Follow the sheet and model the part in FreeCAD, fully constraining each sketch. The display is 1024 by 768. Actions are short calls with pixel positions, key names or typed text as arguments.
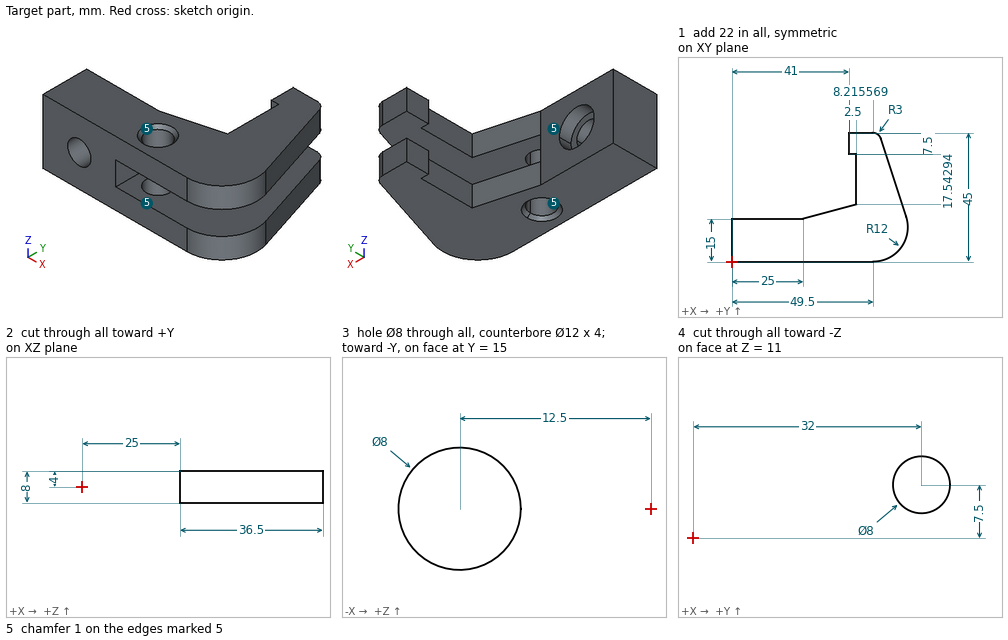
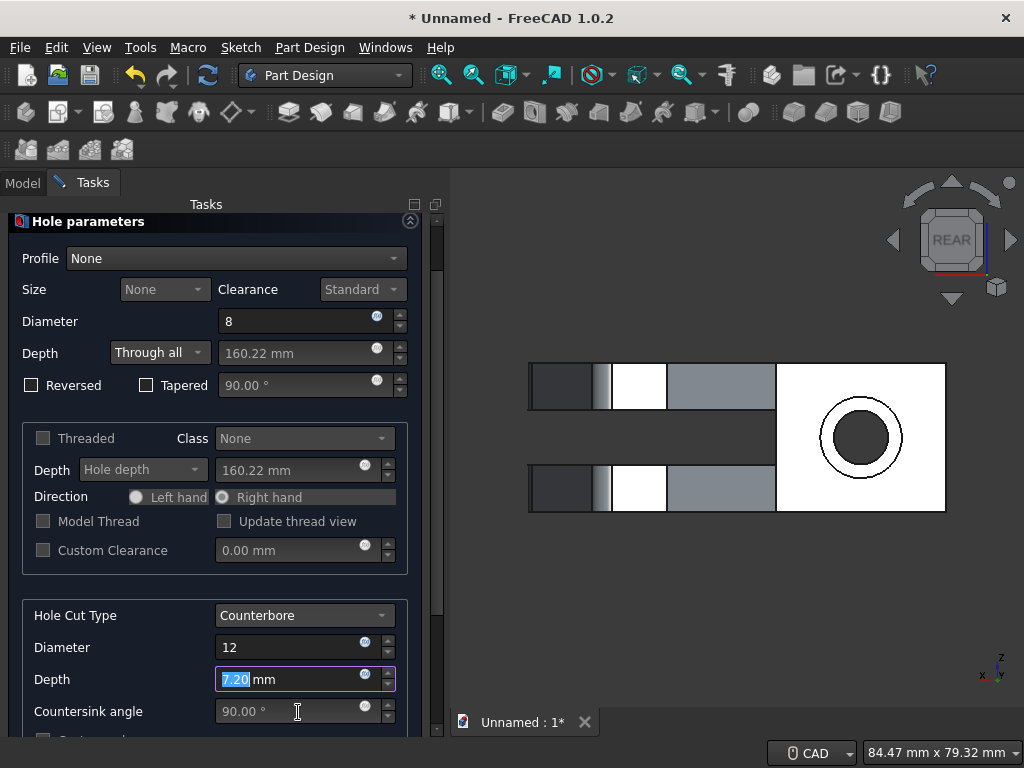
text(4)
key(Tab)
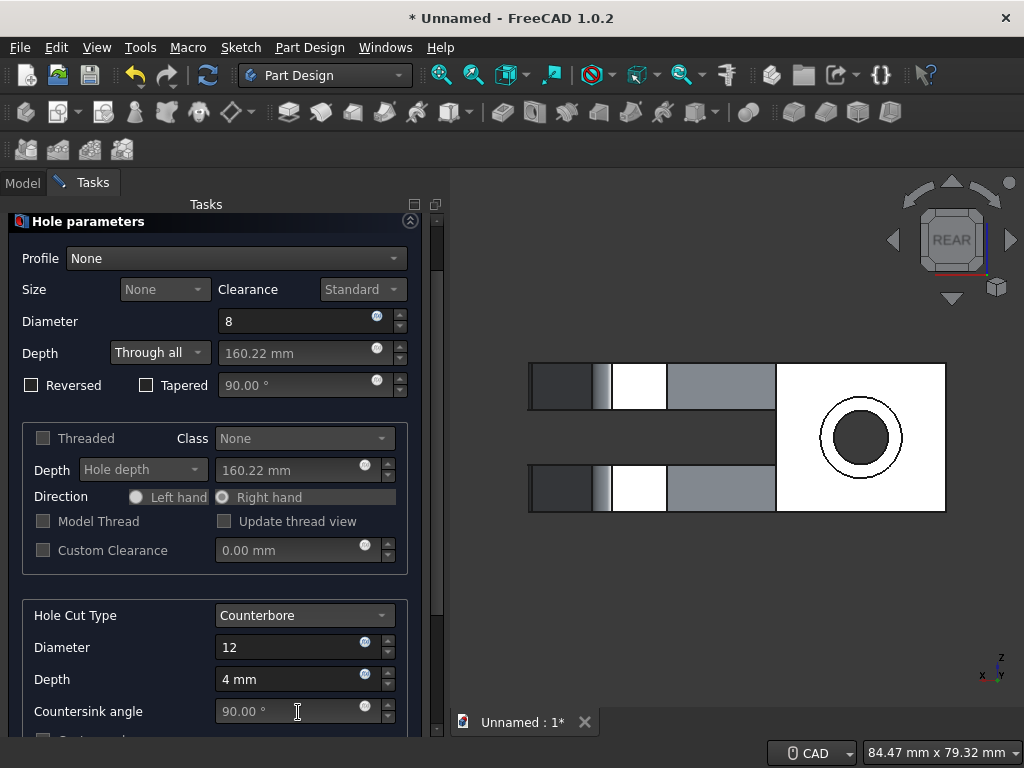
scroll(437, 475, up, 2)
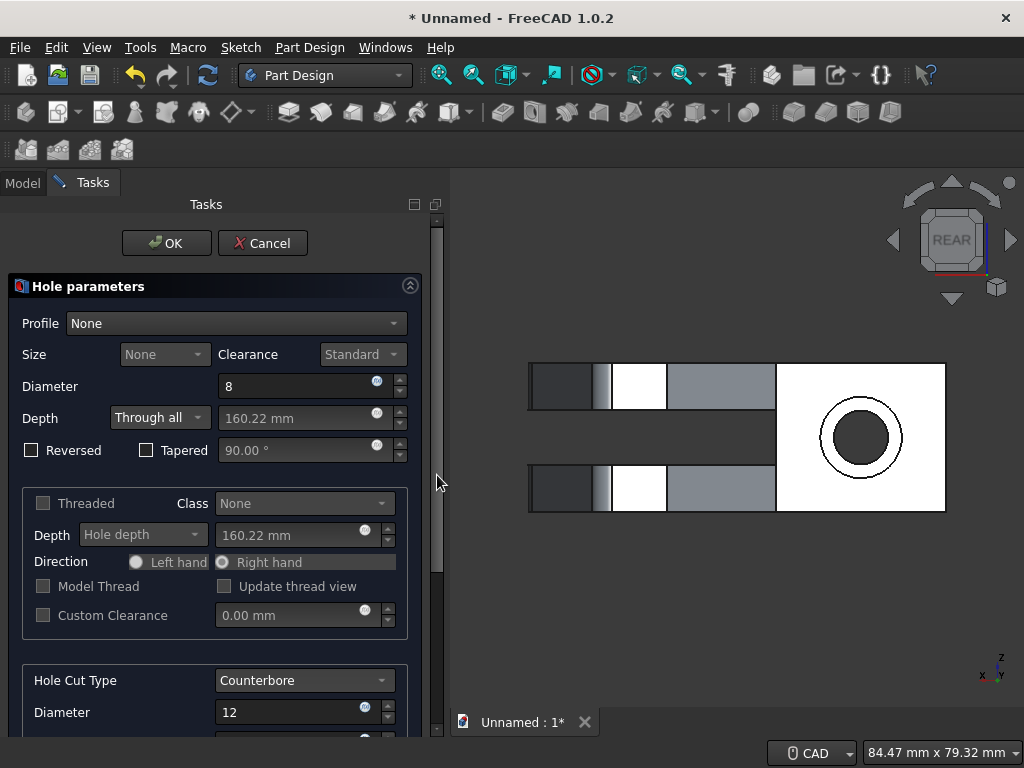
click(167, 243)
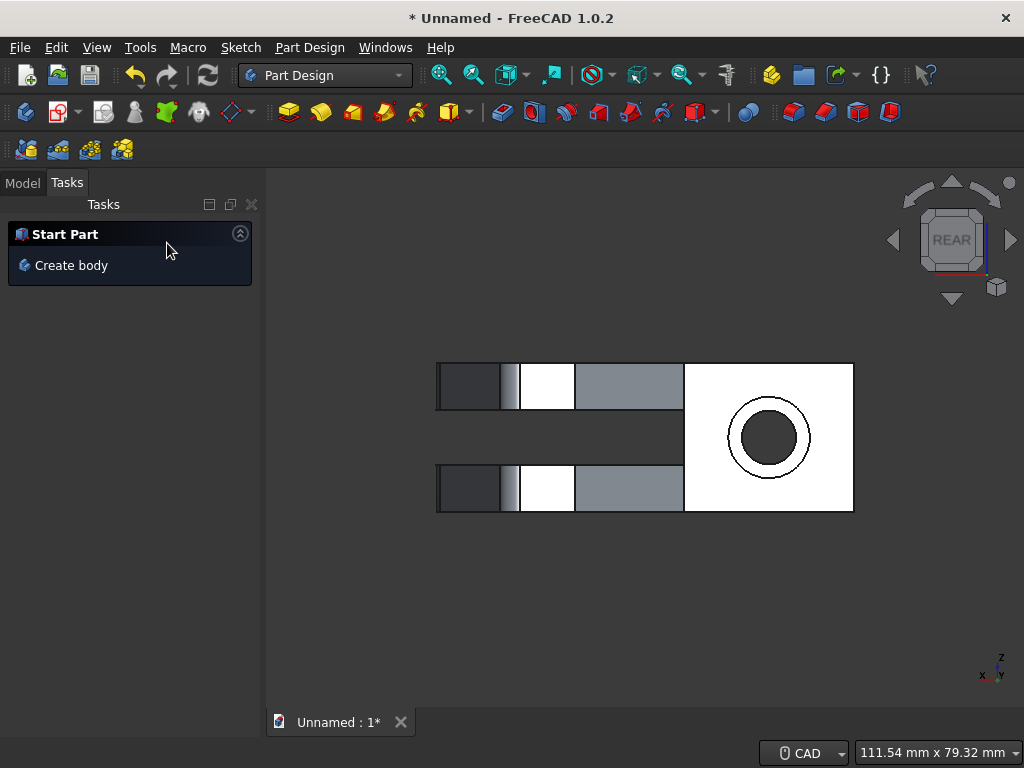
key(0)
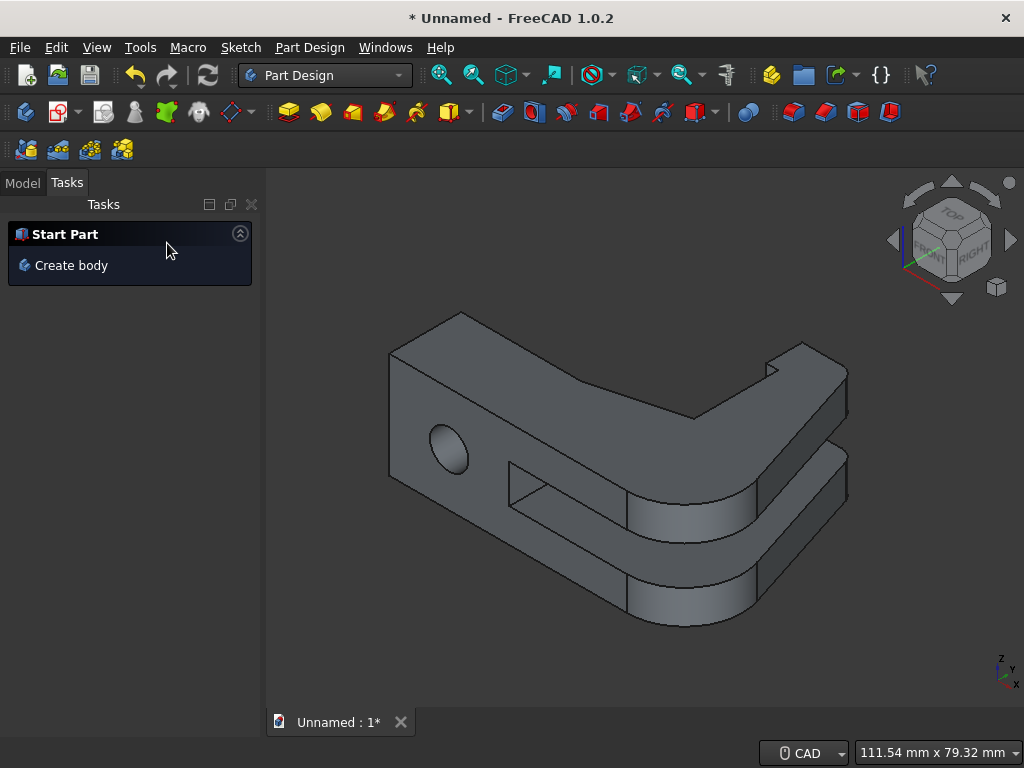
click(668, 460)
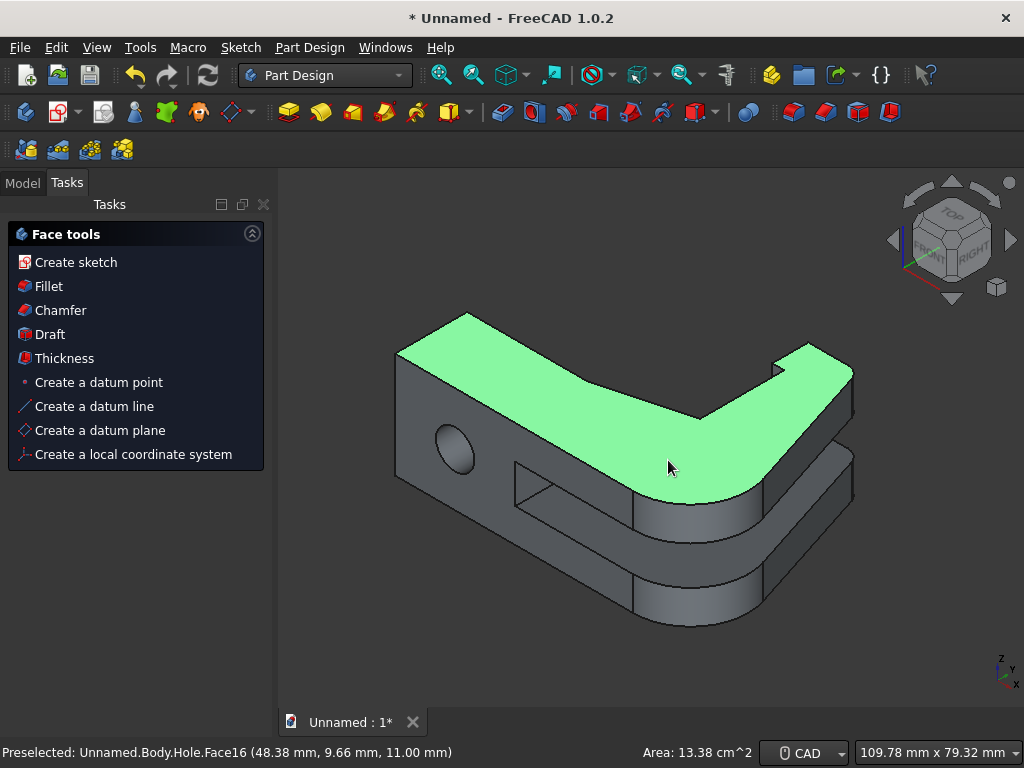
click(58, 112)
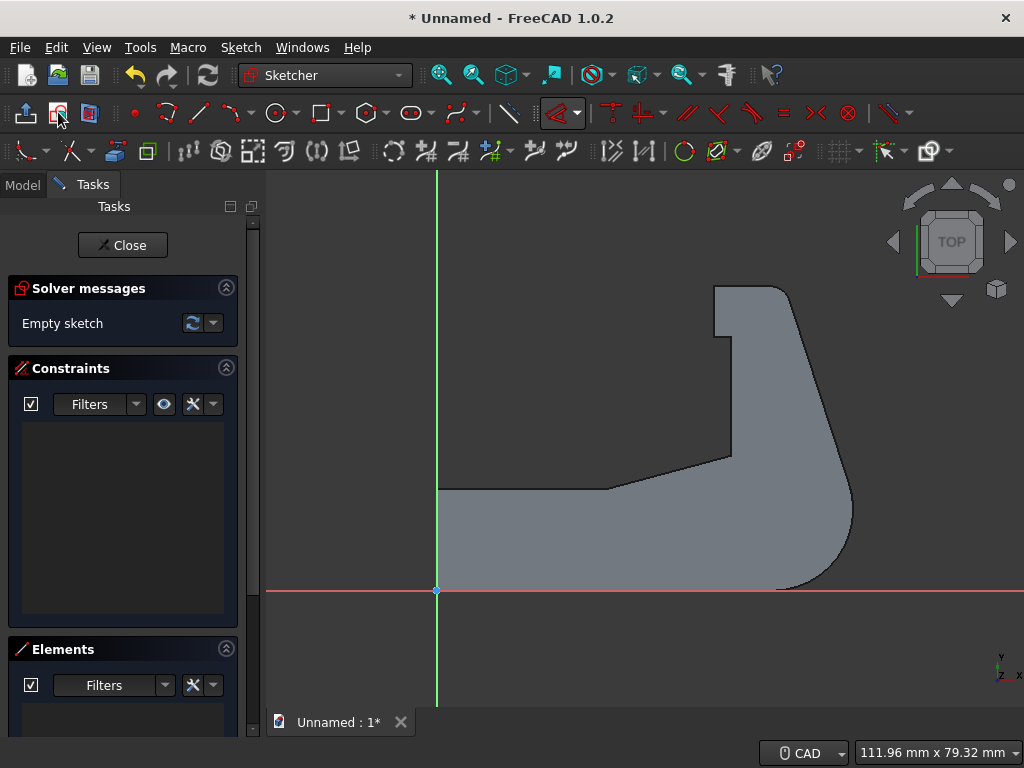
scroll(669, 560, up, 9)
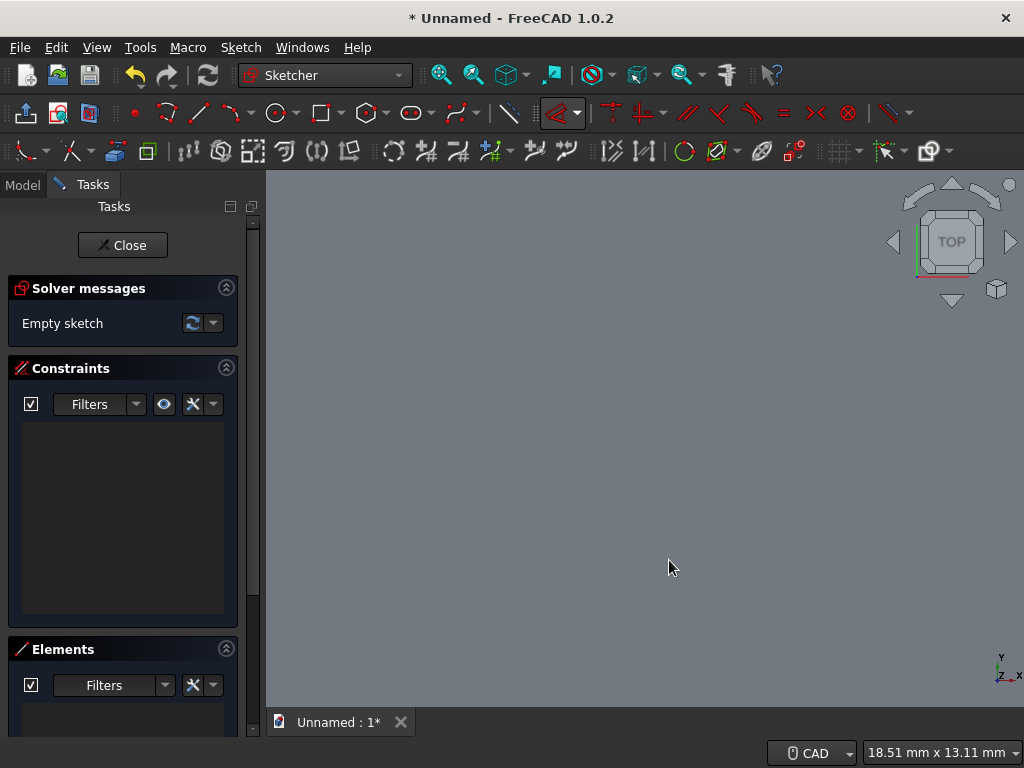
key(g)
key(c)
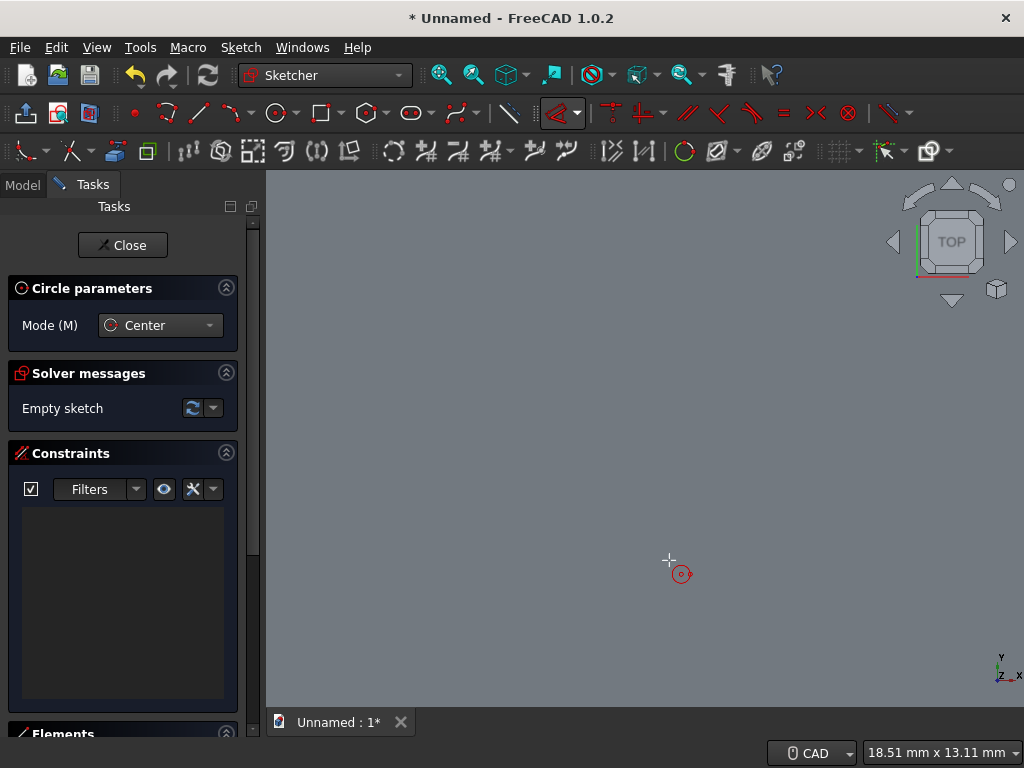
click(572, 436)
click(688, 320)
key(Escape)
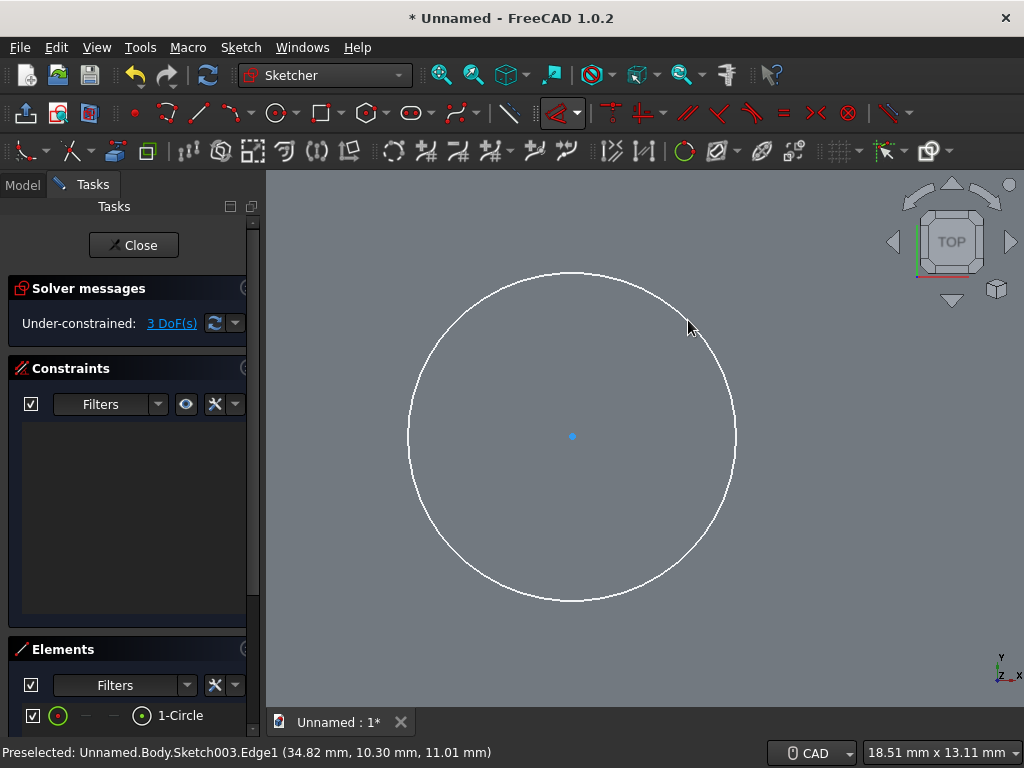
click(688, 321)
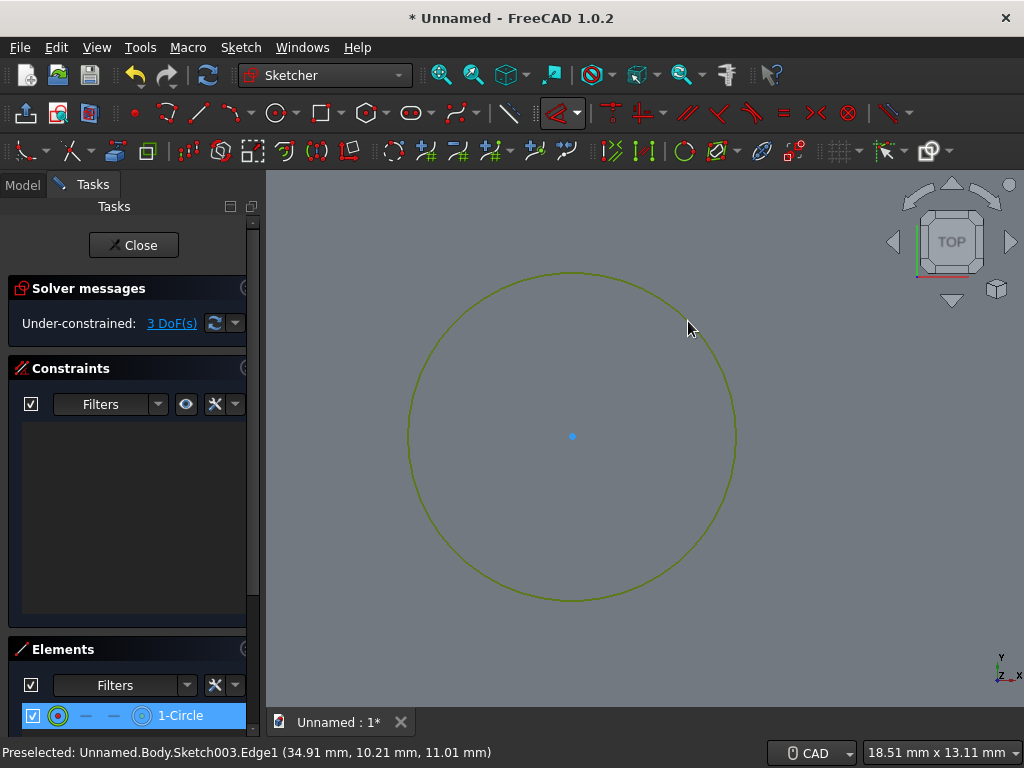
key(k)
key(o)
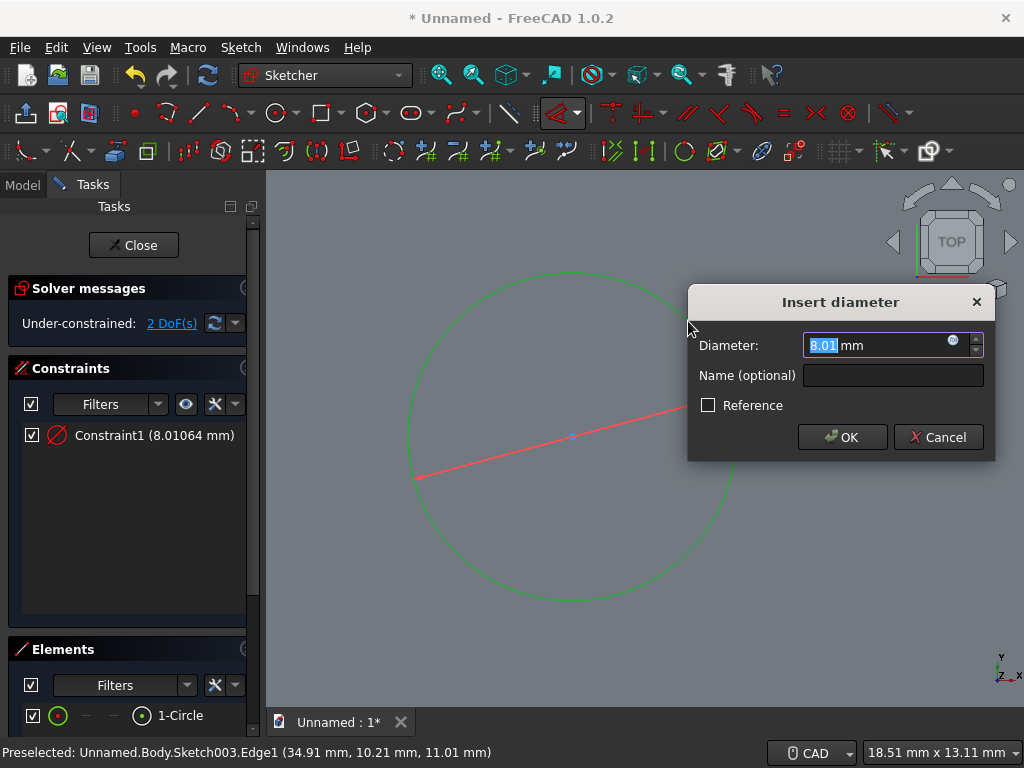
text(8)
key(Return)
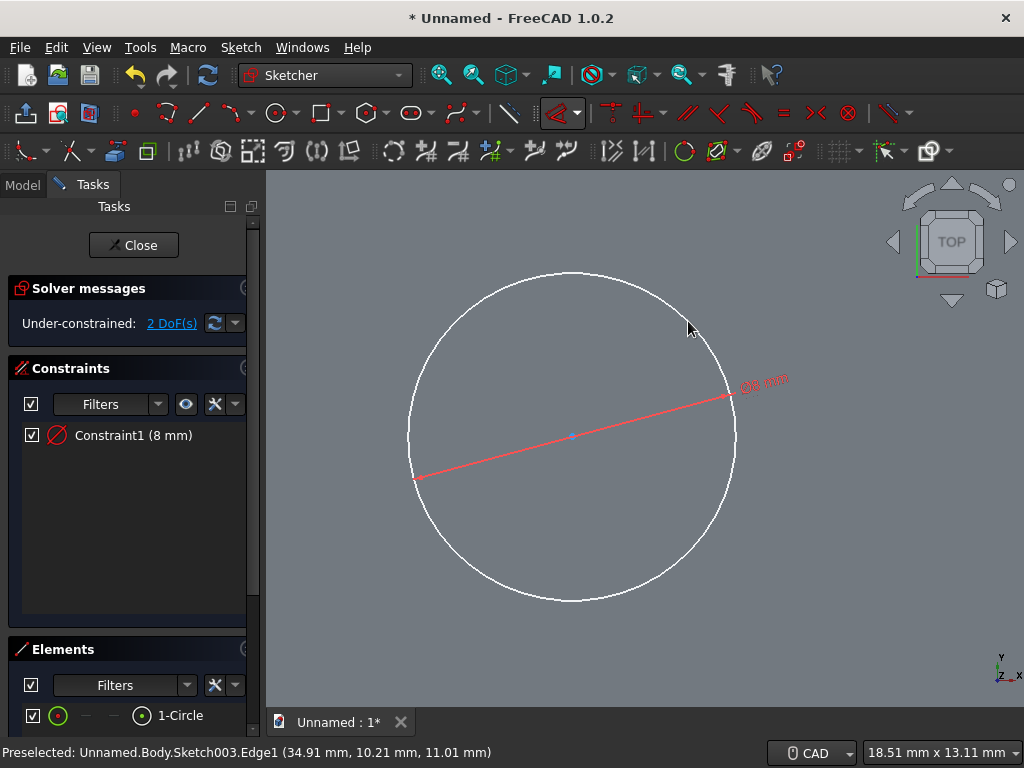
click(572, 437)